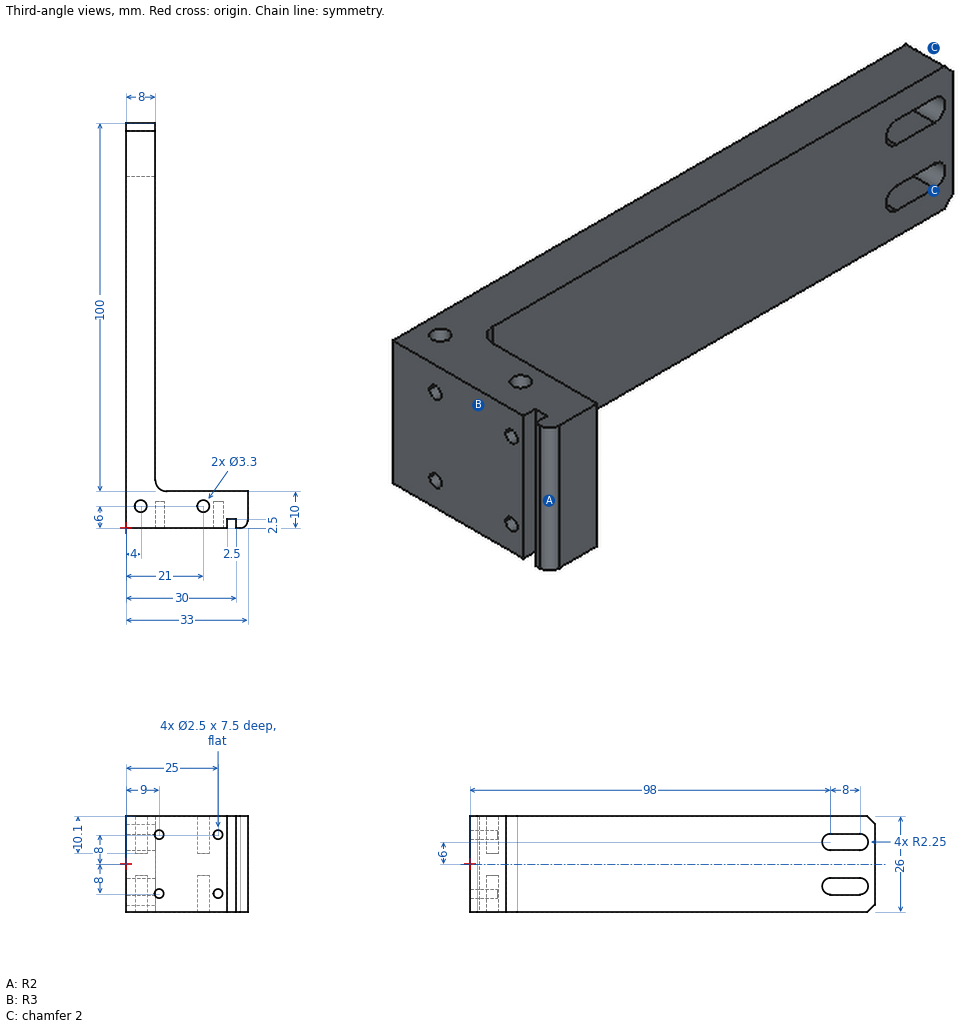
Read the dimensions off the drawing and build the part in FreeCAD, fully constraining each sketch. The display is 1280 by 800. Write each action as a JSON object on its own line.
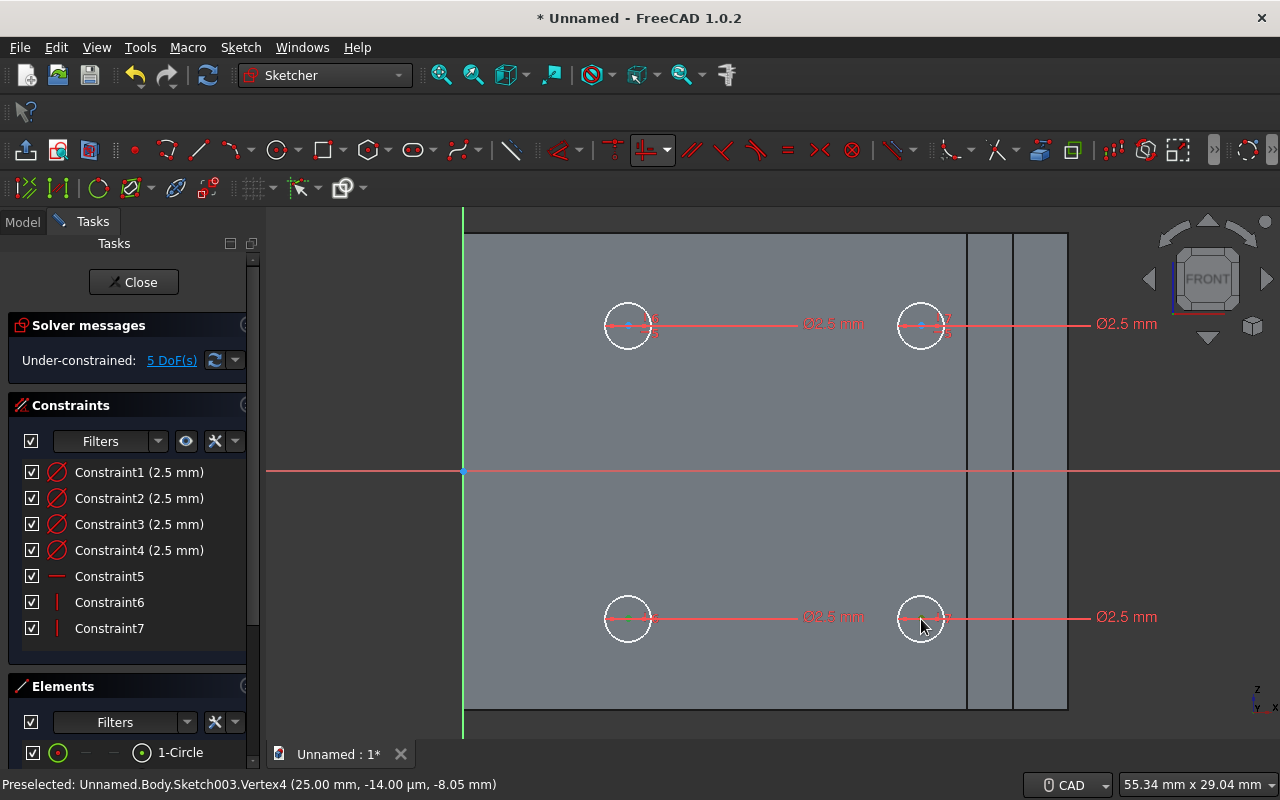
{"action": "key", "text": "h"}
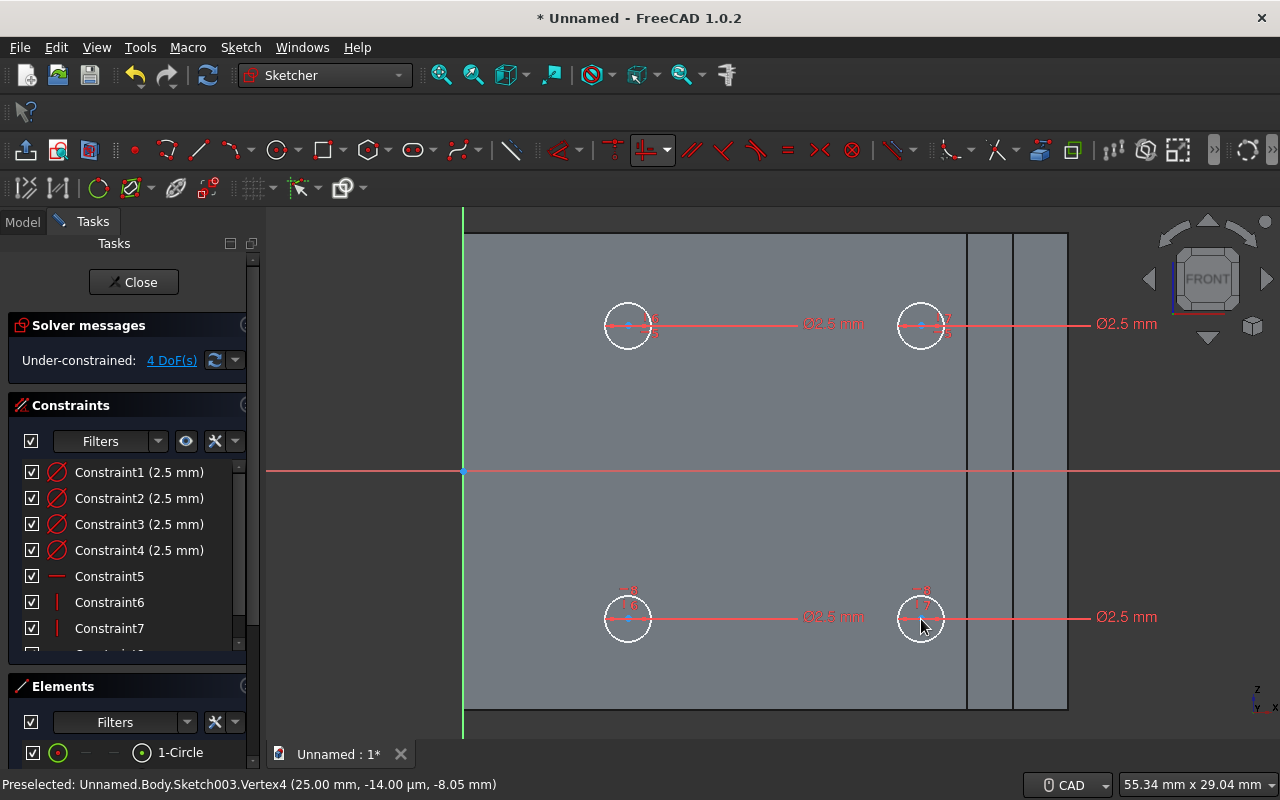
{"action": "left_click", "coordinate": [558, 150]}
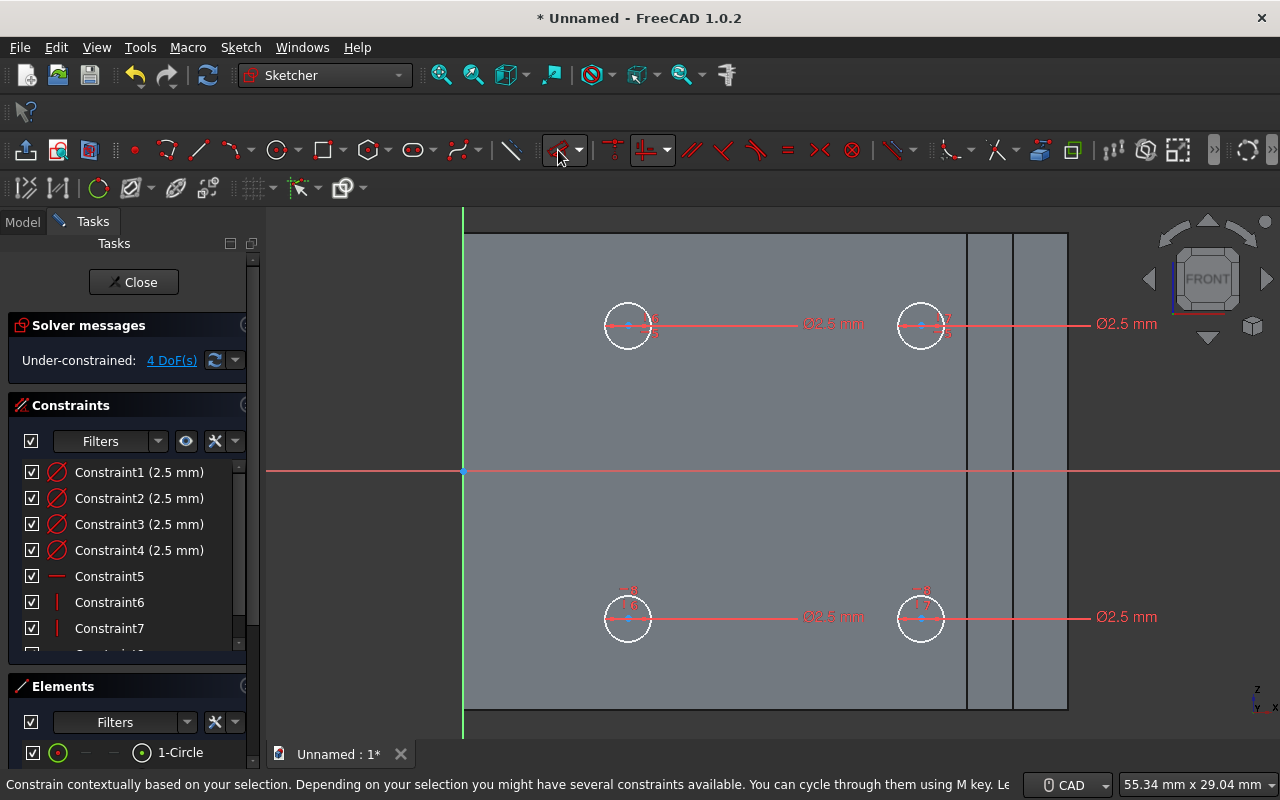
{"action": "left_click", "coordinate": [921, 326]}
{"action": "left_click", "coordinate": [429, 399]}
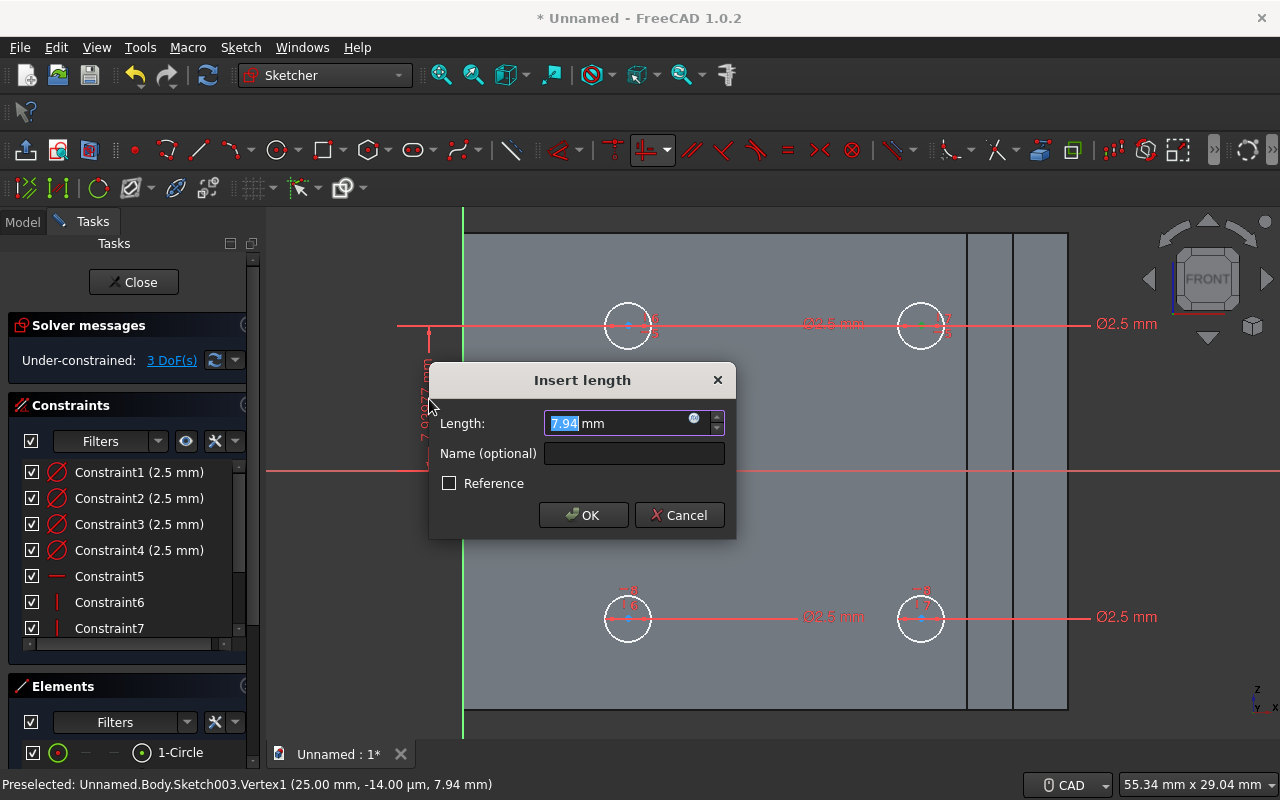
{"action": "type", "text": "8"}
{"action": "key", "text": "Return"}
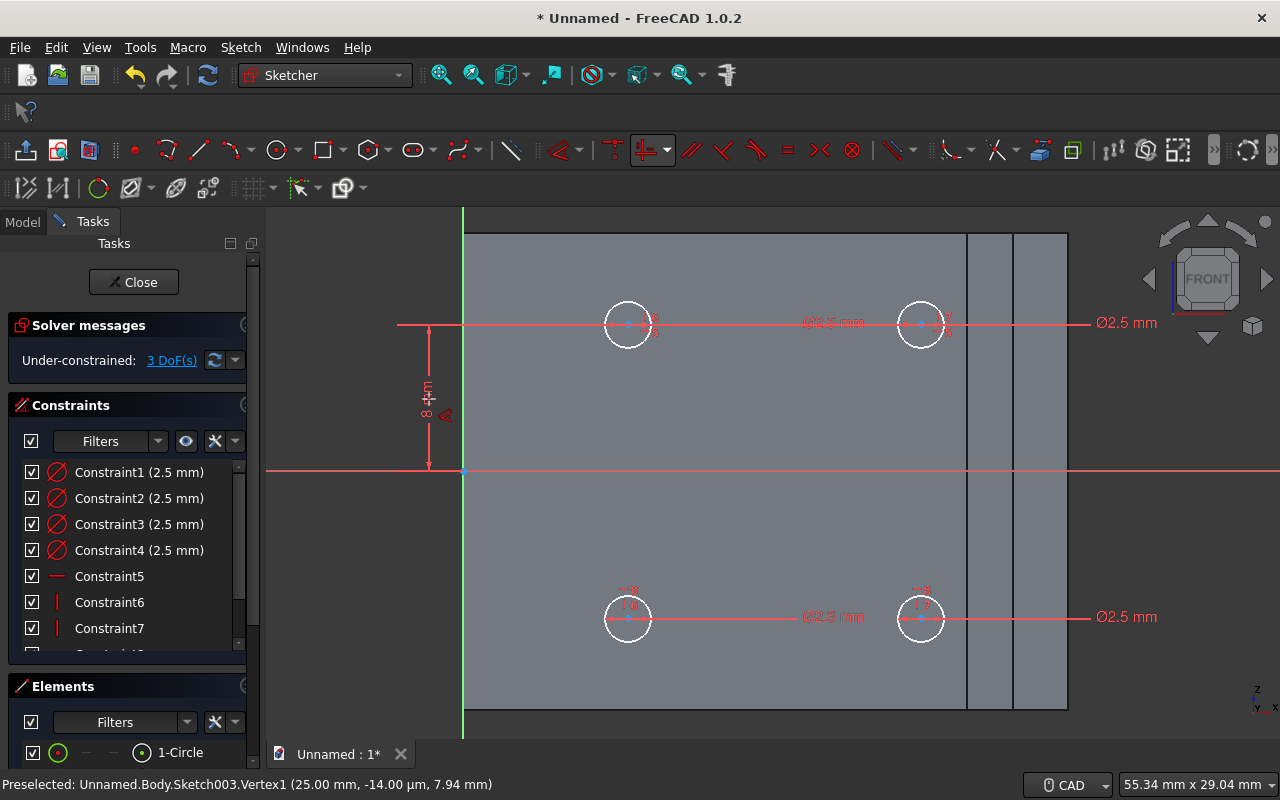
{"action": "left_click", "coordinate": [628, 325]}
{"action": "left_click", "coordinate": [546, 291]}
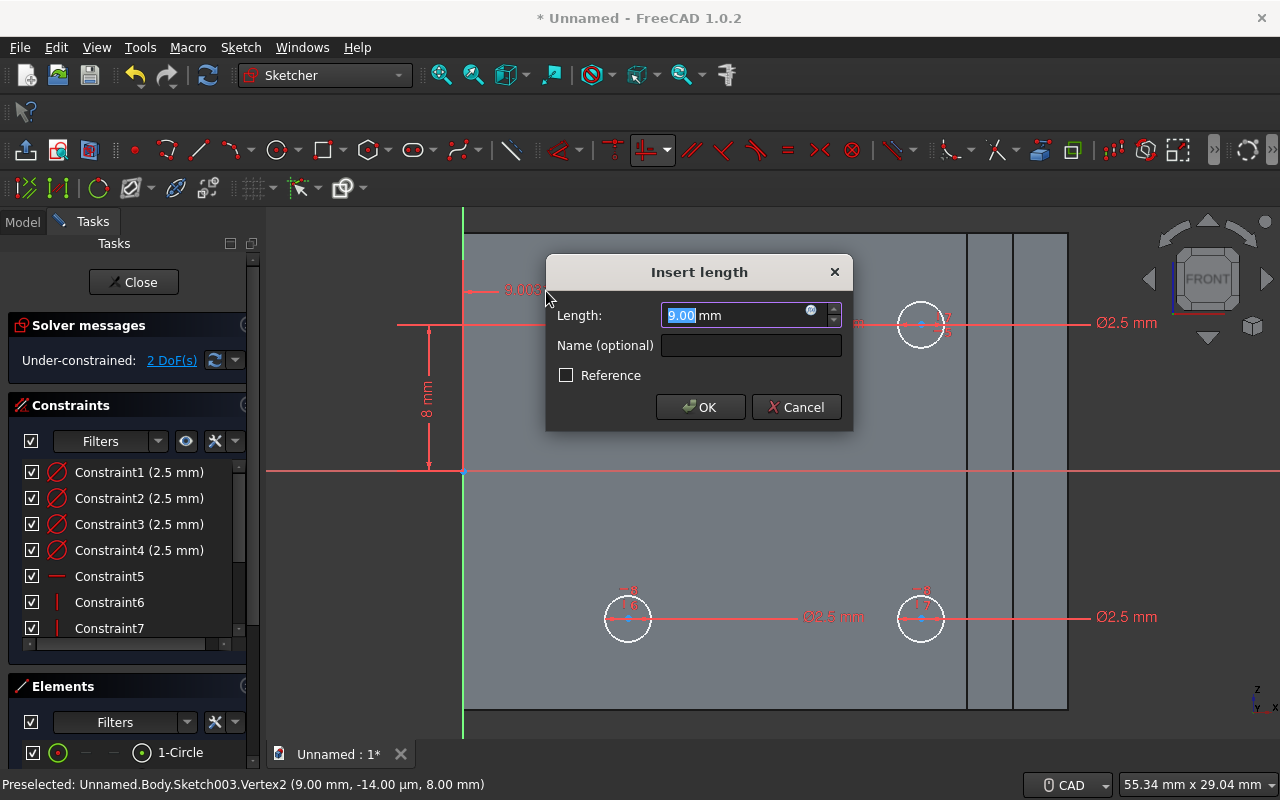
{"action": "type", "text": "9"}
{"action": "key", "text": "Return"}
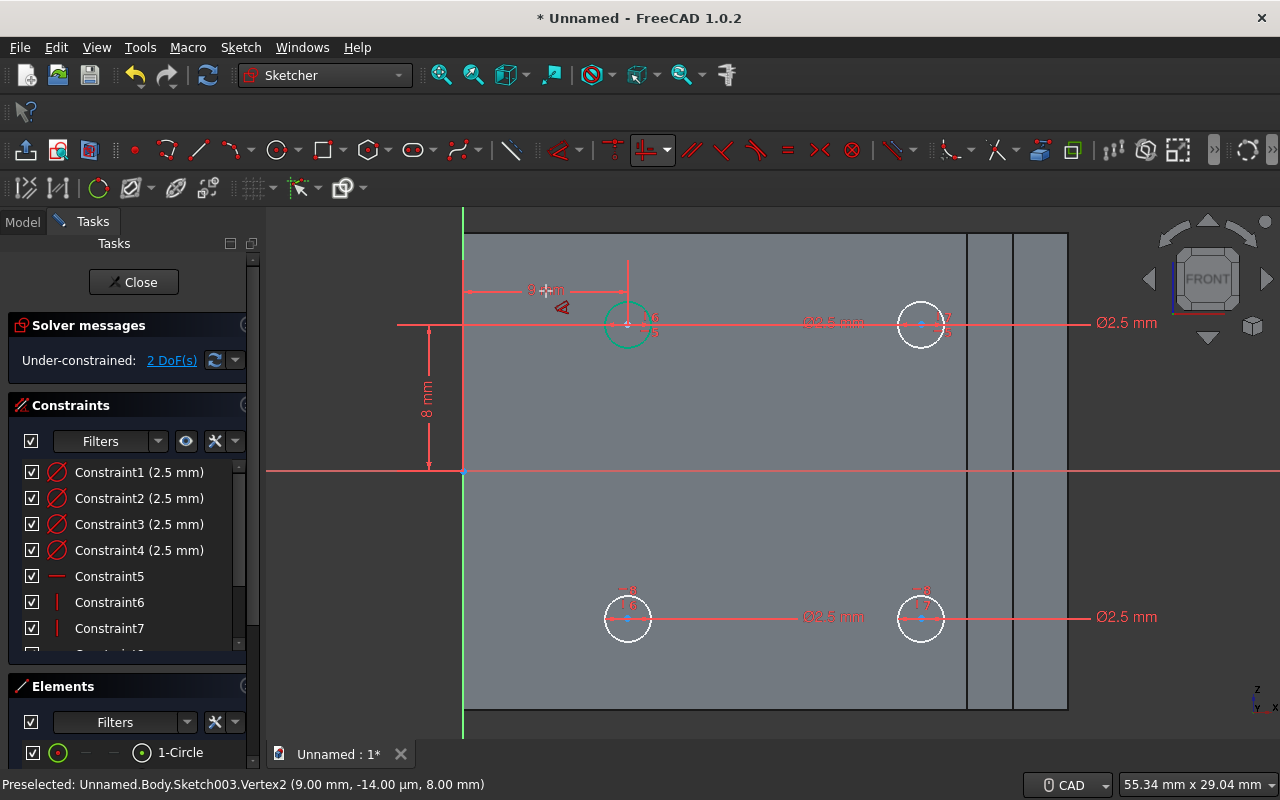
{"action": "left_click", "coordinate": [628, 619]}
{"action": "left_click", "coordinate": [429, 545]}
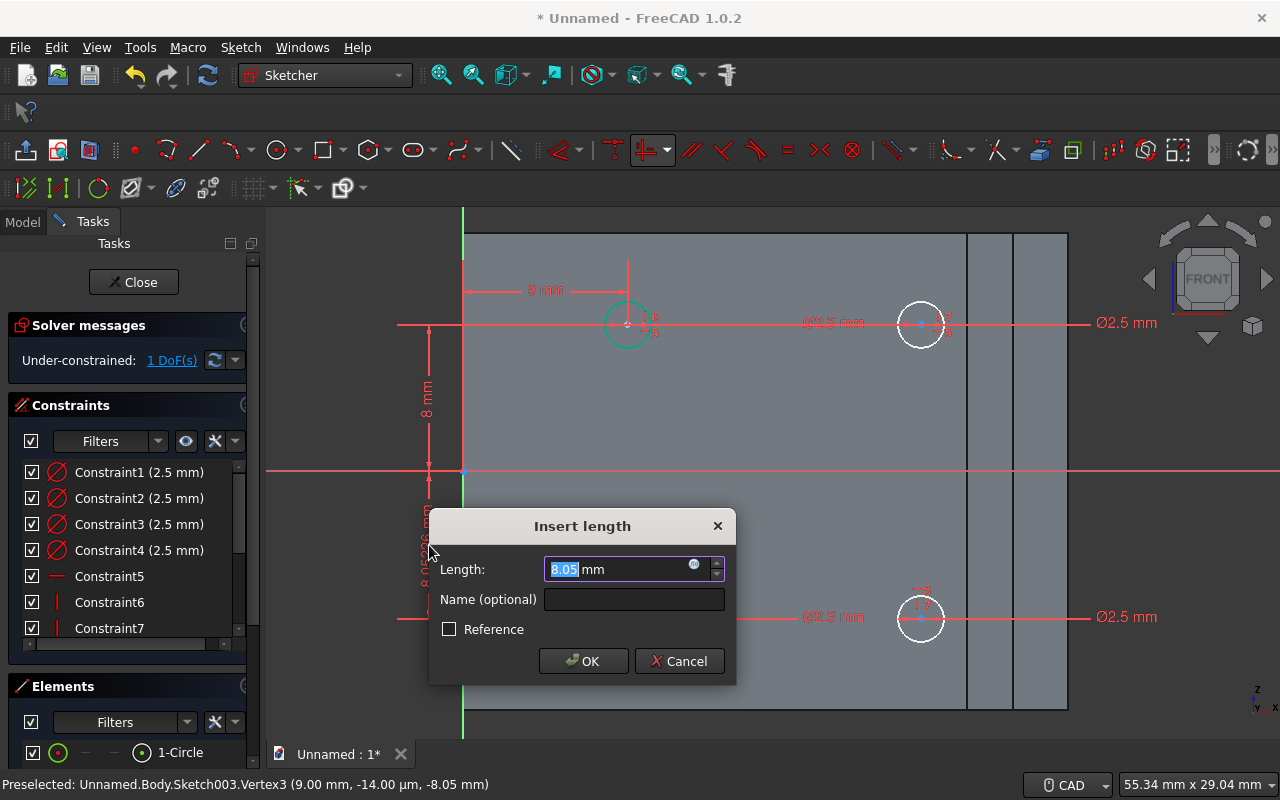
{"action": "type", "text": "8"}
{"action": "key", "text": "Return"}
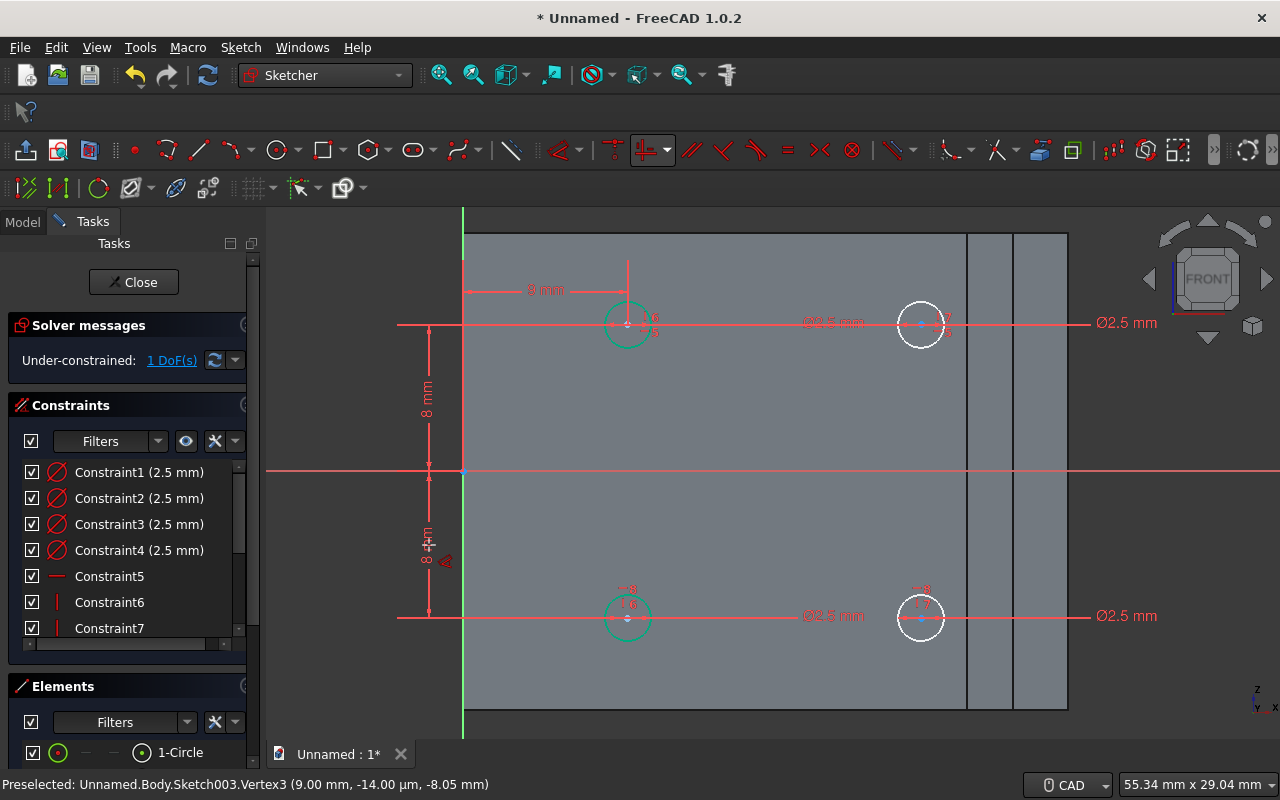
{"action": "left_click", "coordinate": [921, 325]}
{"action": "left_click", "coordinate": [692, 291]}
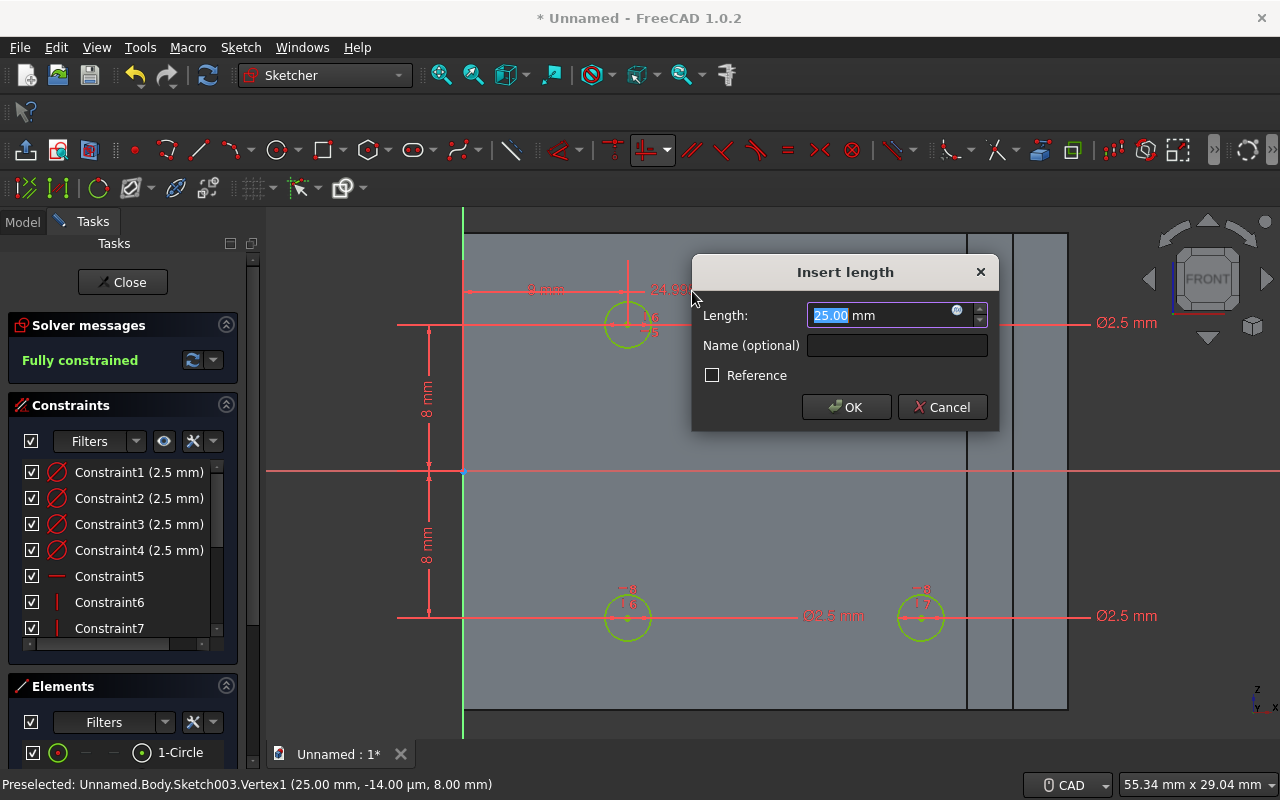
{"action": "type", "text": "25"}
{"action": "key", "text": "Return"}
{"action": "key", "text": "Escape"}